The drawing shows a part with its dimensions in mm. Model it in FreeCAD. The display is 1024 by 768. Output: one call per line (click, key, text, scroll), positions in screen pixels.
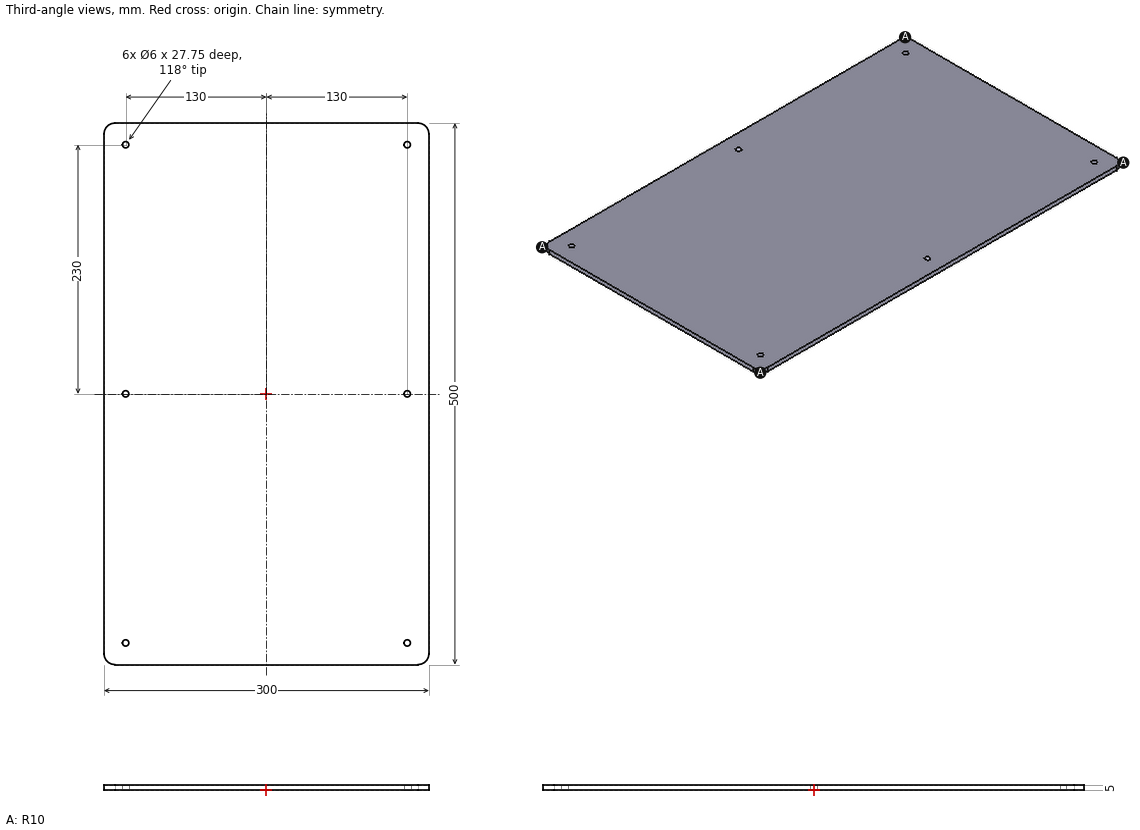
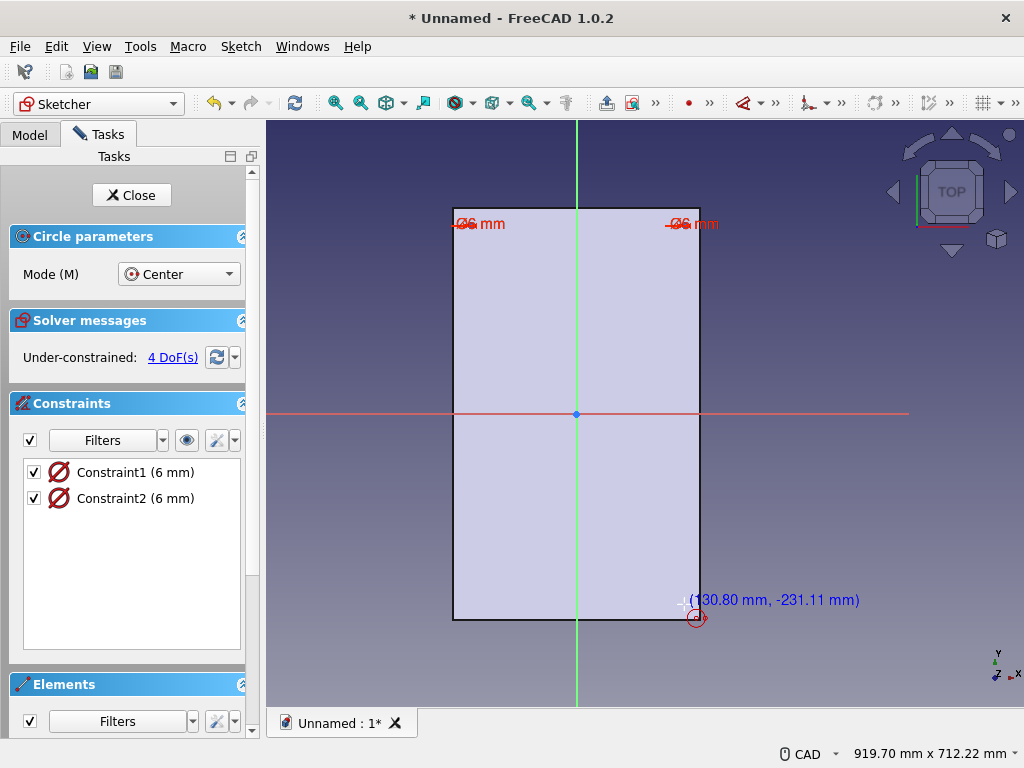
click(684, 604)
move(686, 602)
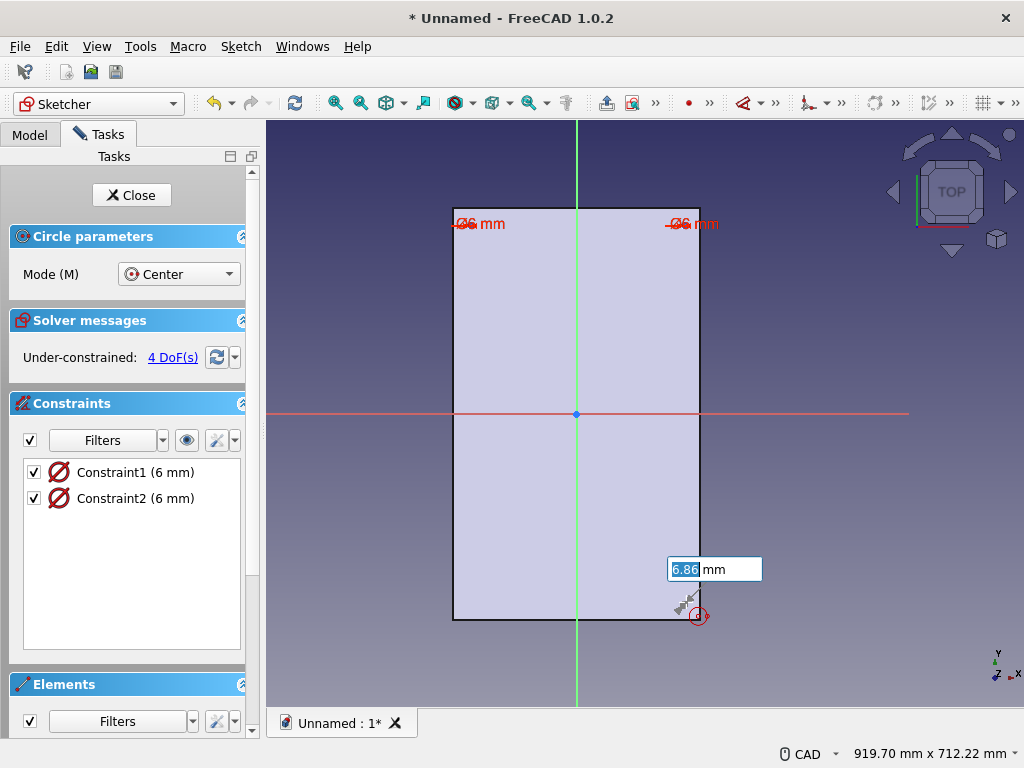
text(6)
key(Return)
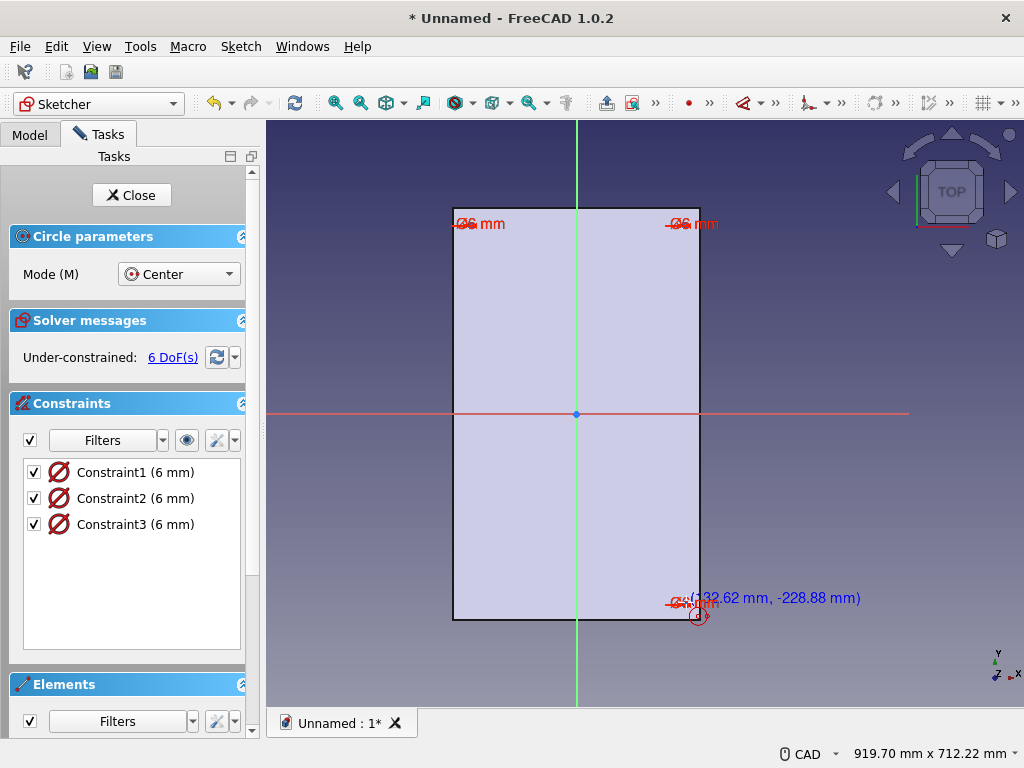
scroll(470, 604, up, 12)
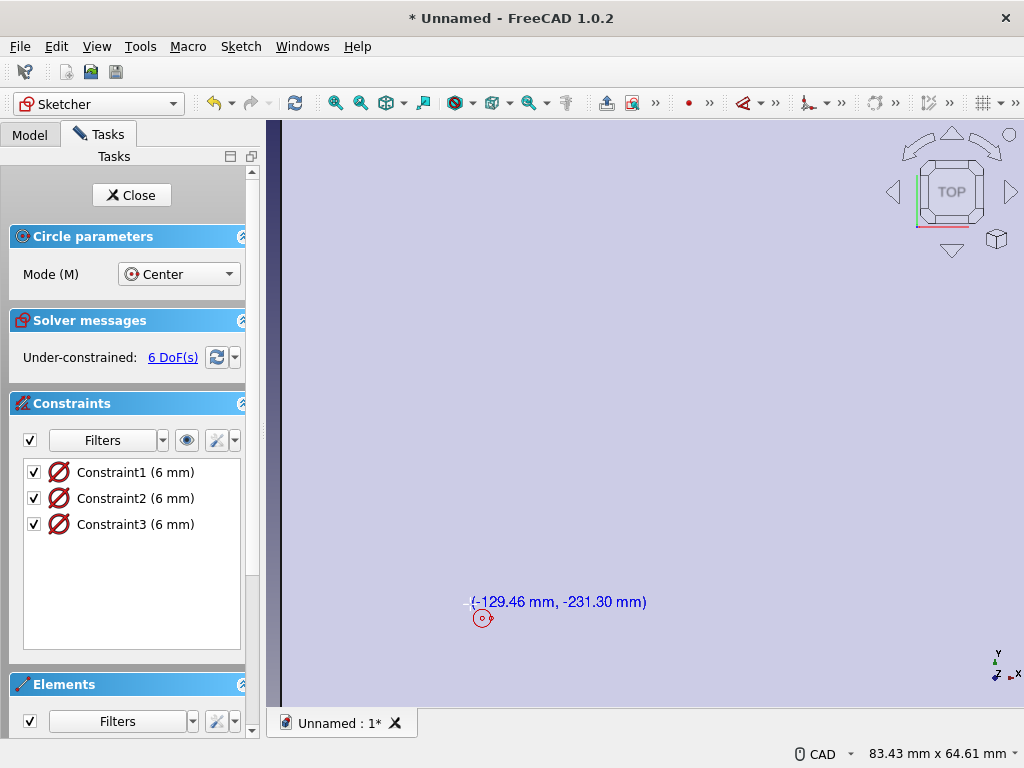
scroll(470, 604, down, 12)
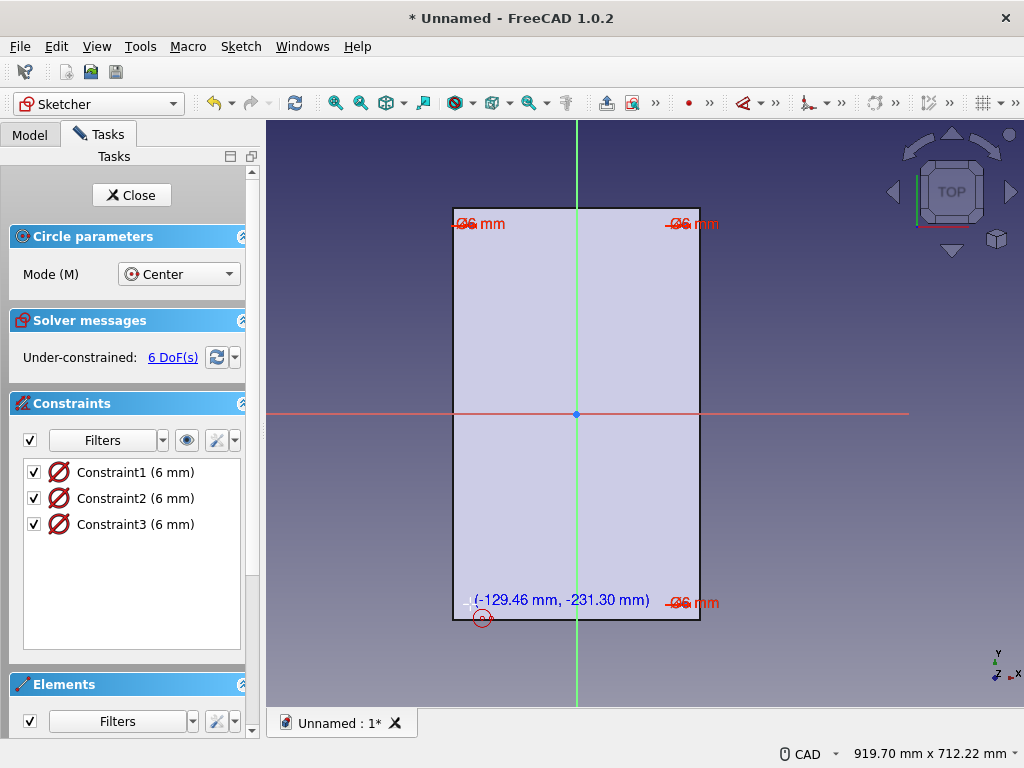
click(470, 604)
move(471, 602)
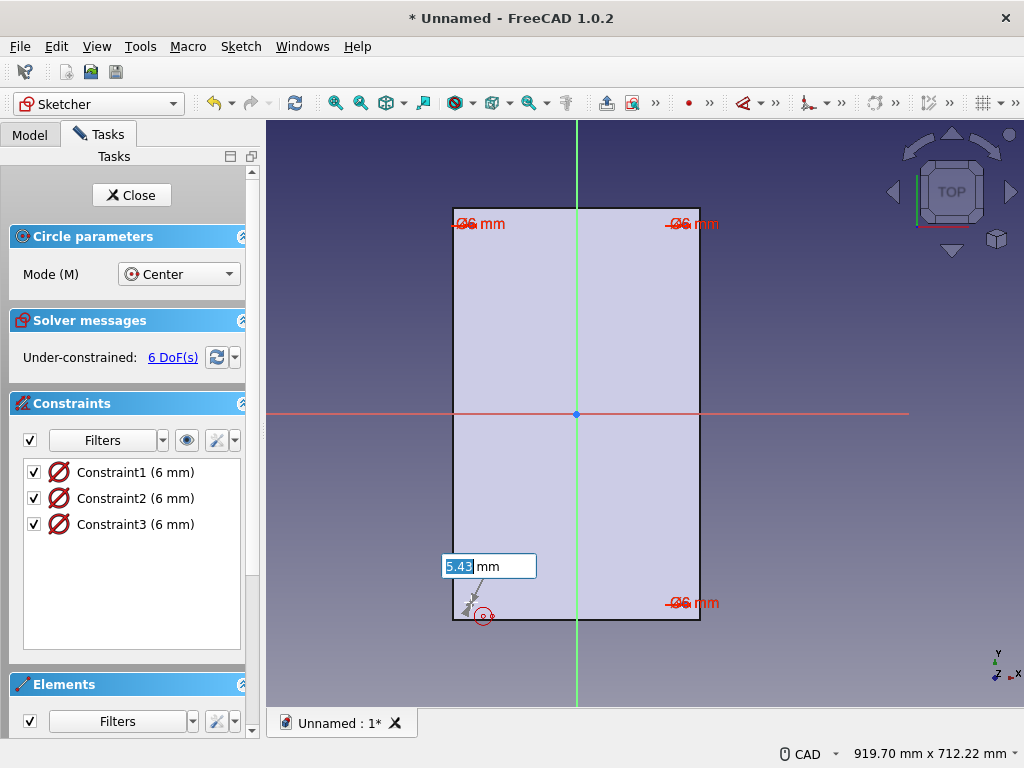
text(6)
key(Return)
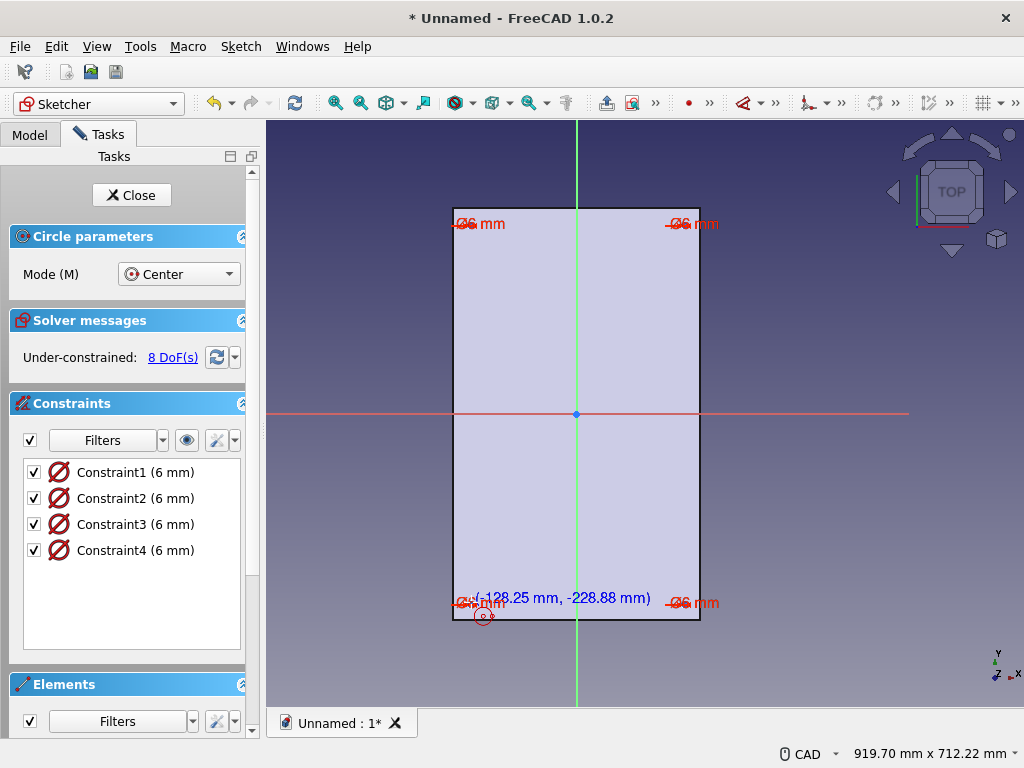
scroll(470, 414, up, 12)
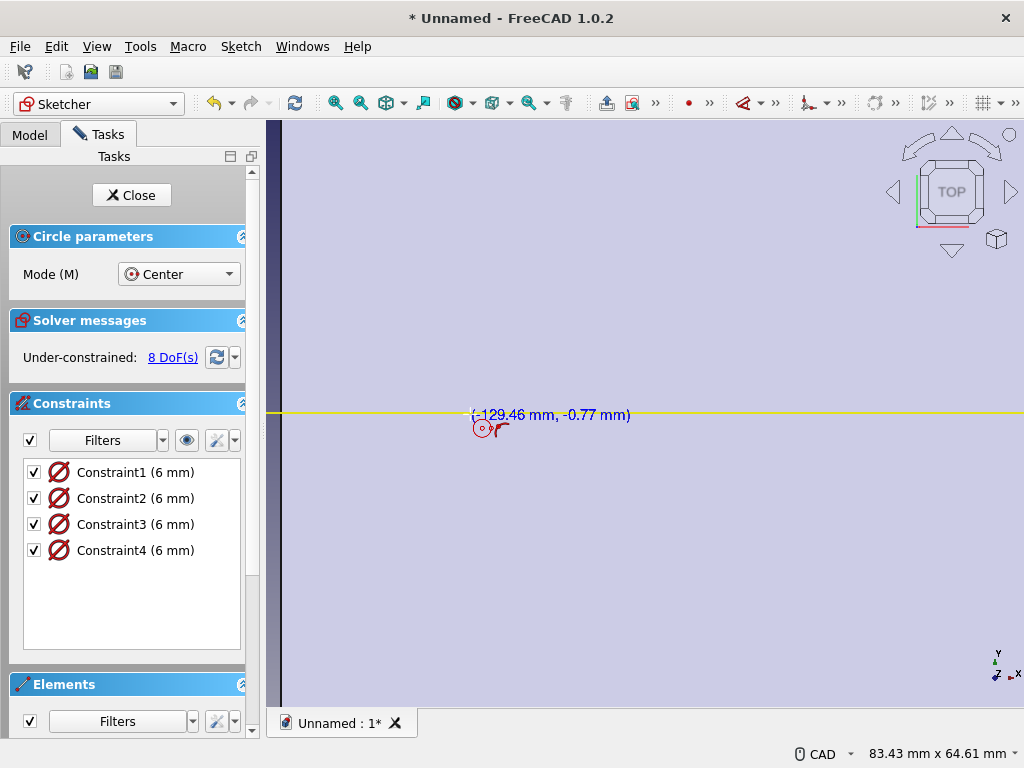
scroll(470, 414, down, 12)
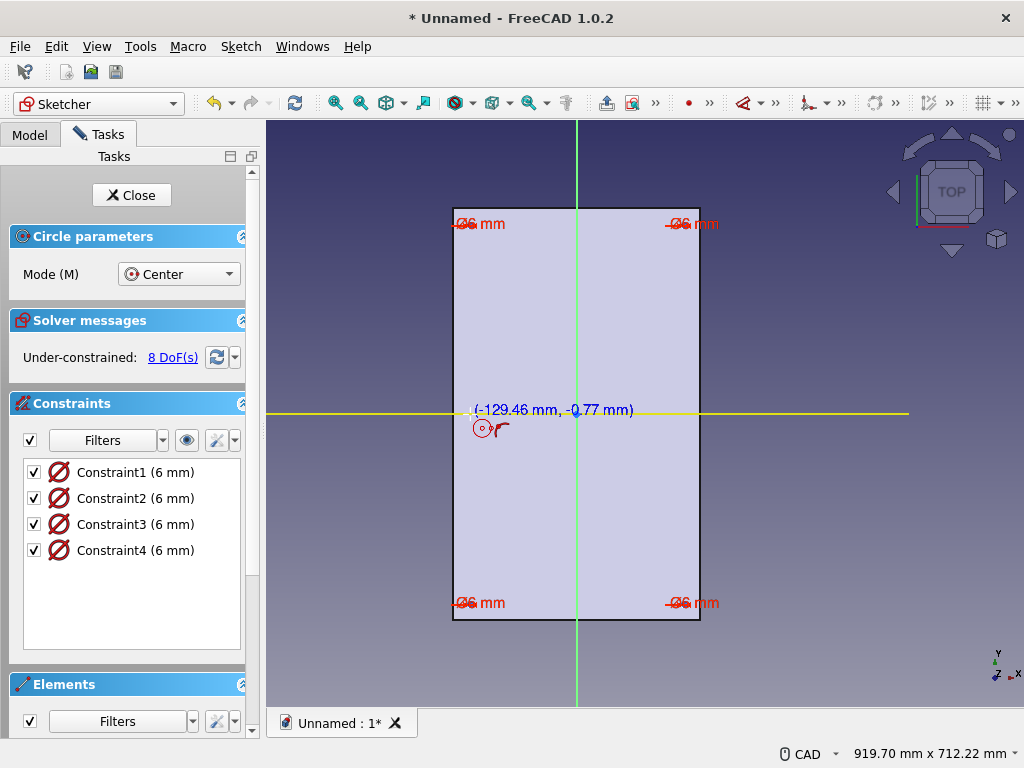
click(470, 414)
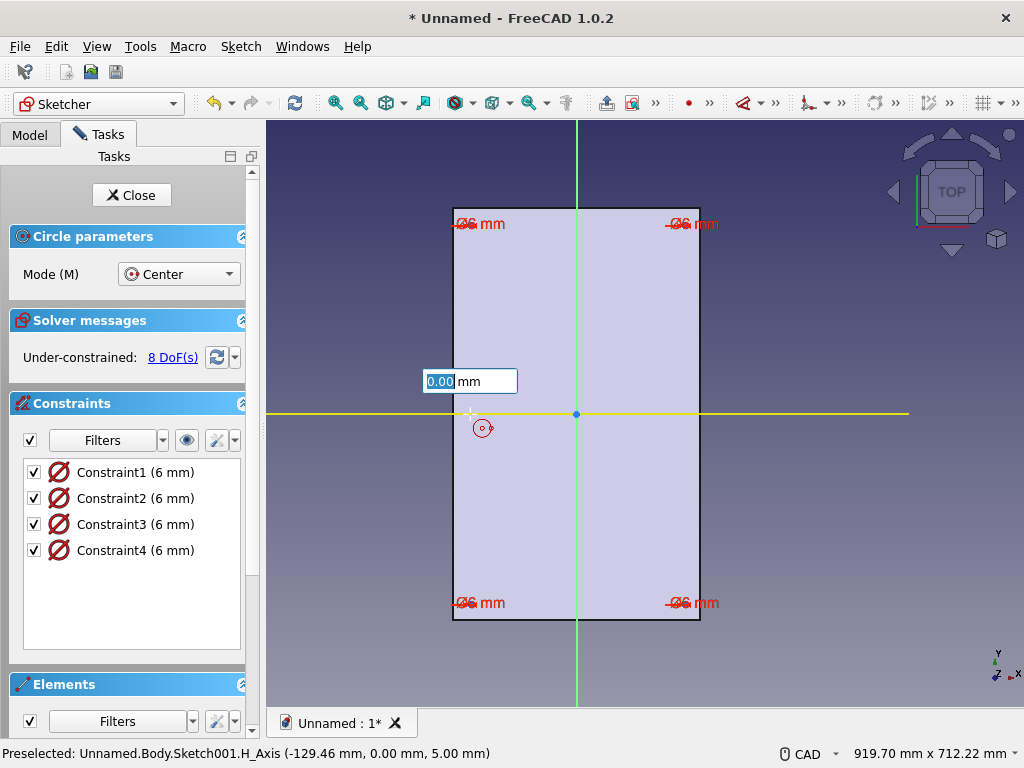
scroll(469, 417, up, 10)
move(465, 411)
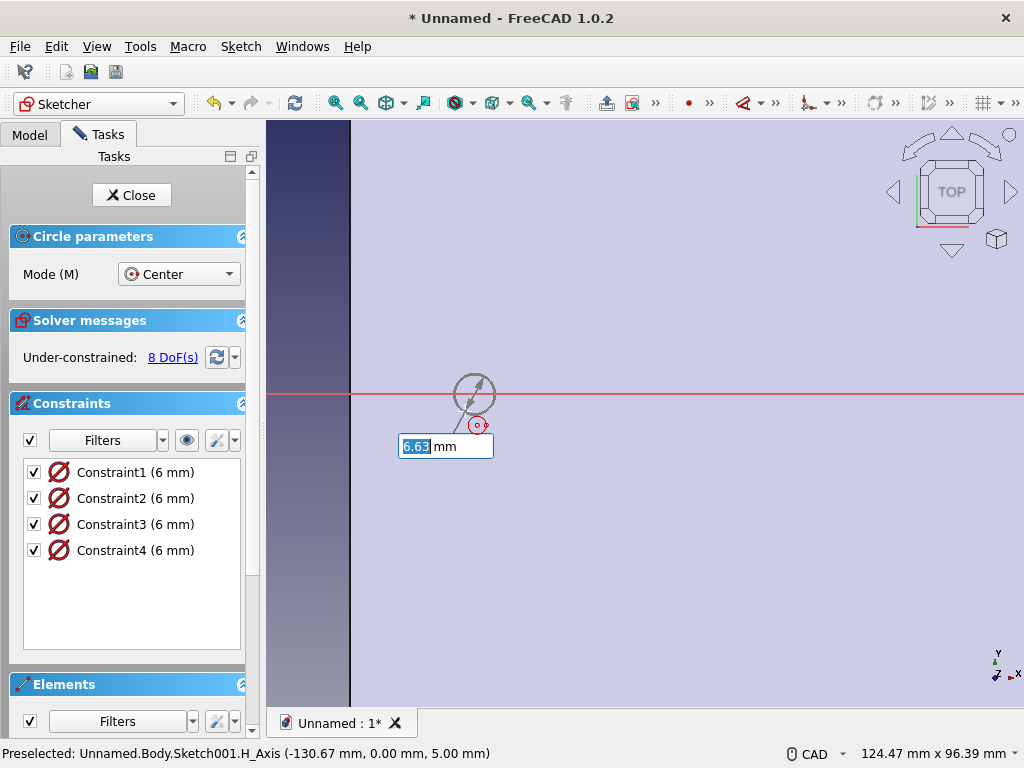
text(6)
key(Return)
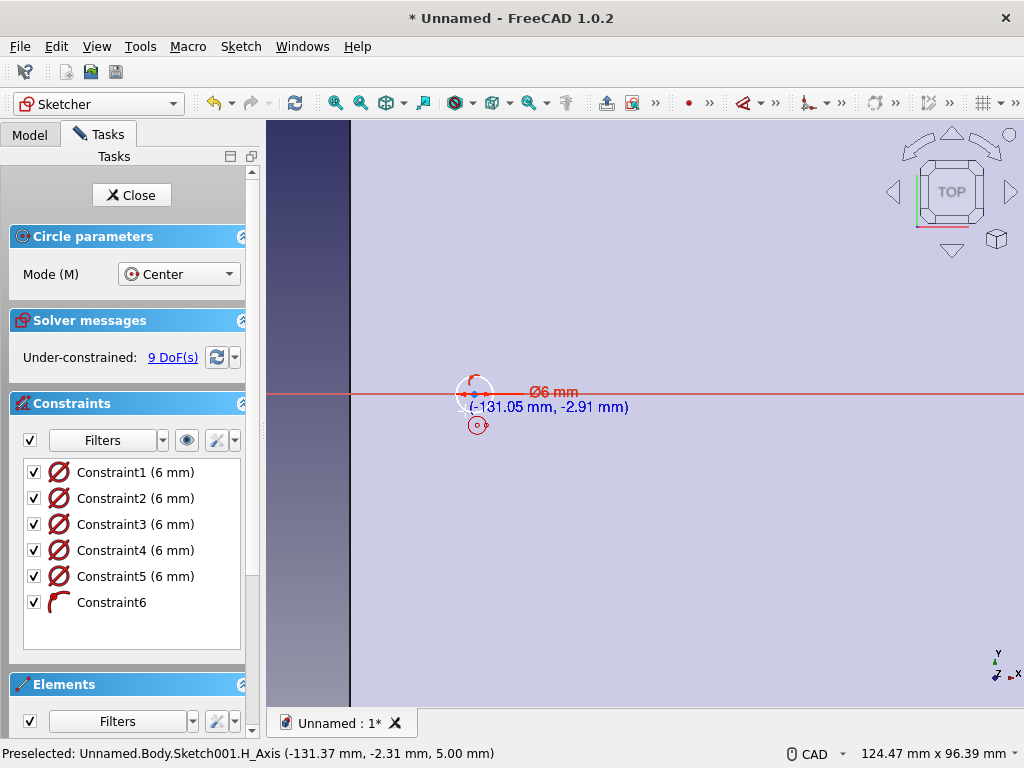
scroll(469, 417, down, 10)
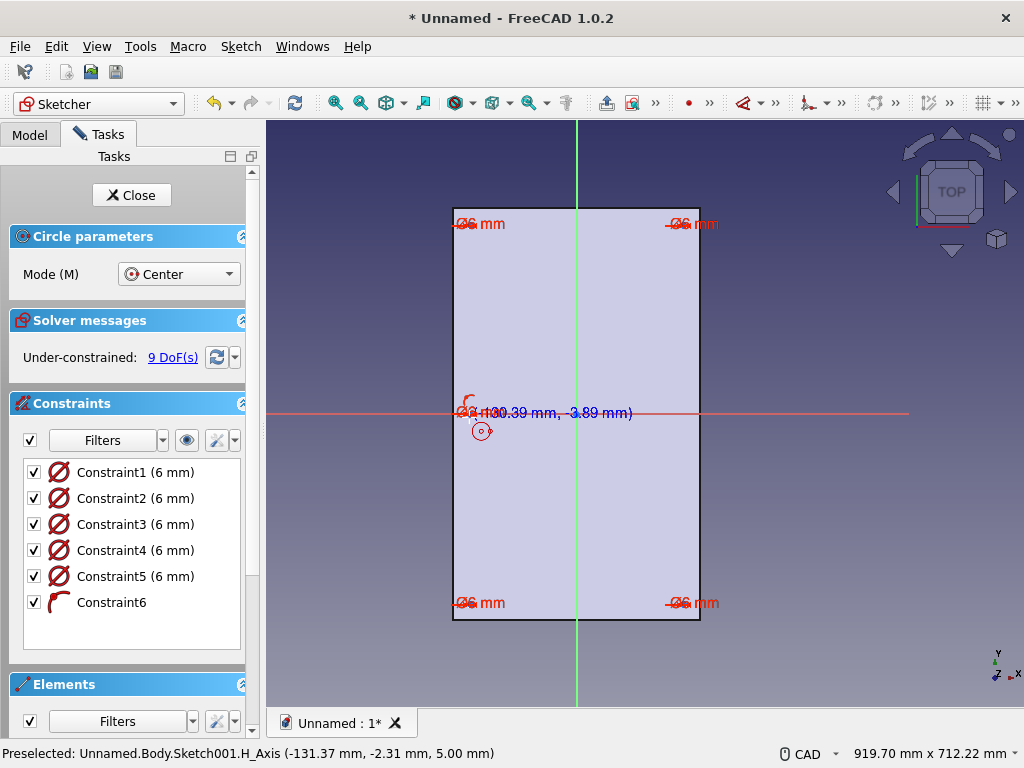
scroll(684, 414, up, 12)